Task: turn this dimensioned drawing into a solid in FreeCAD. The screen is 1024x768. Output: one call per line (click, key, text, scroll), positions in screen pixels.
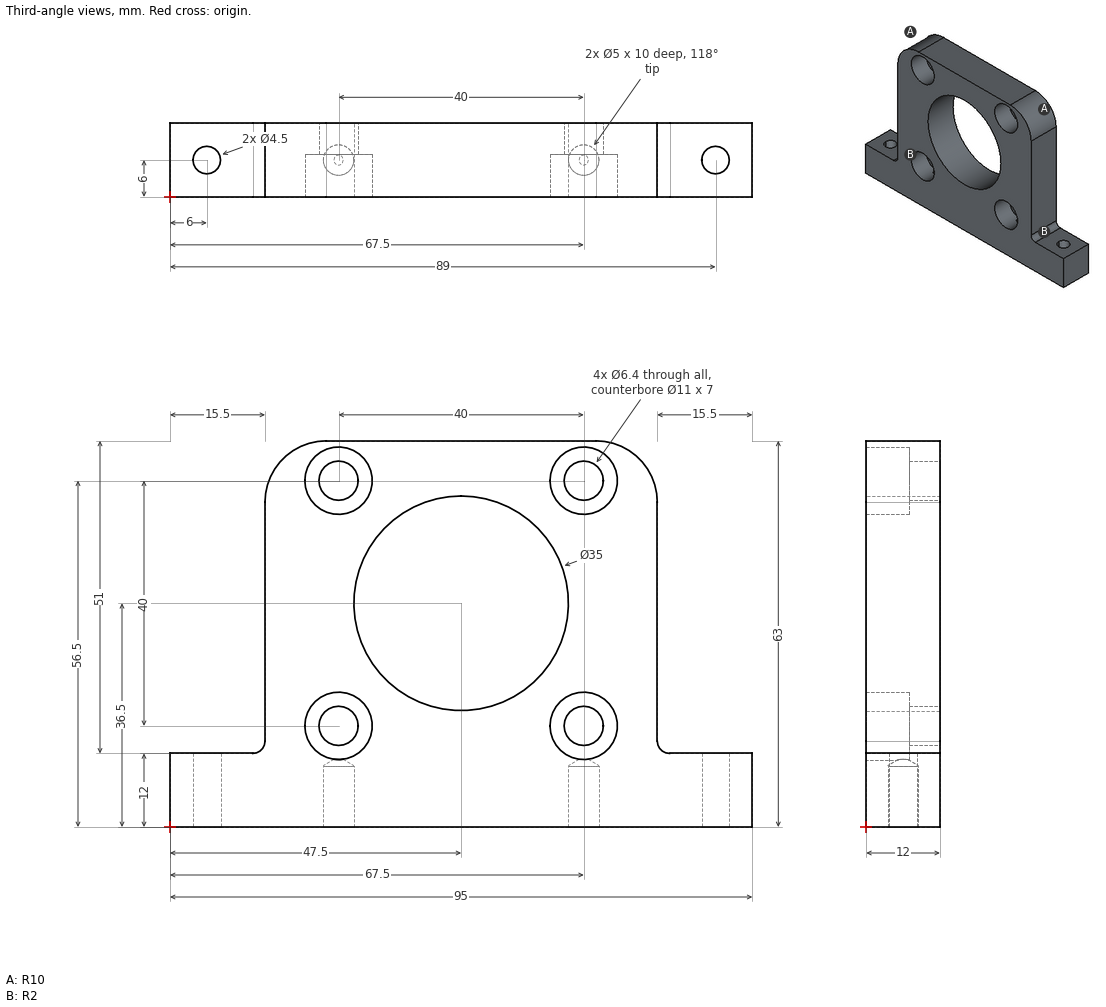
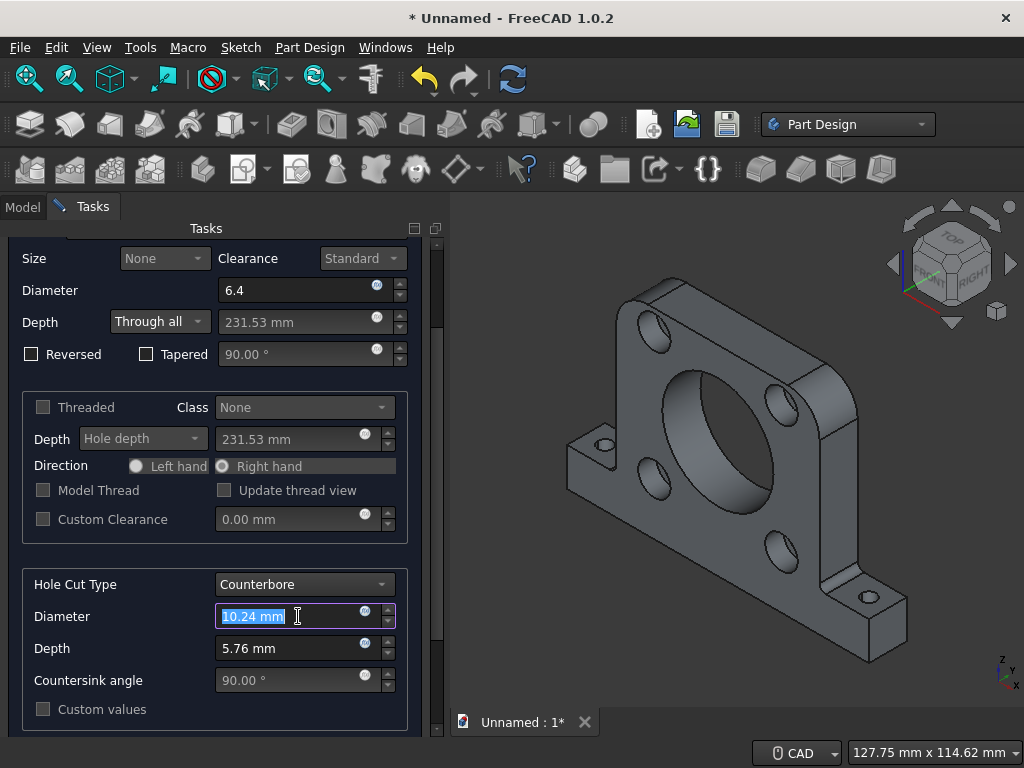
text(11)
key(Tab)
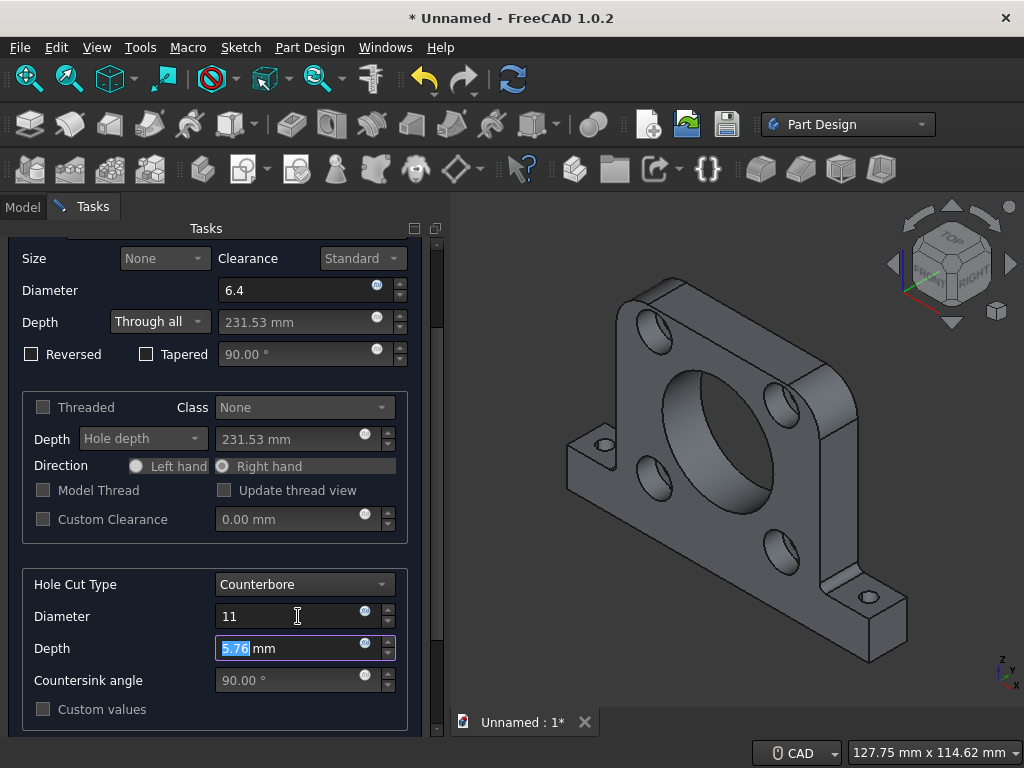
text(7)
key(Tab)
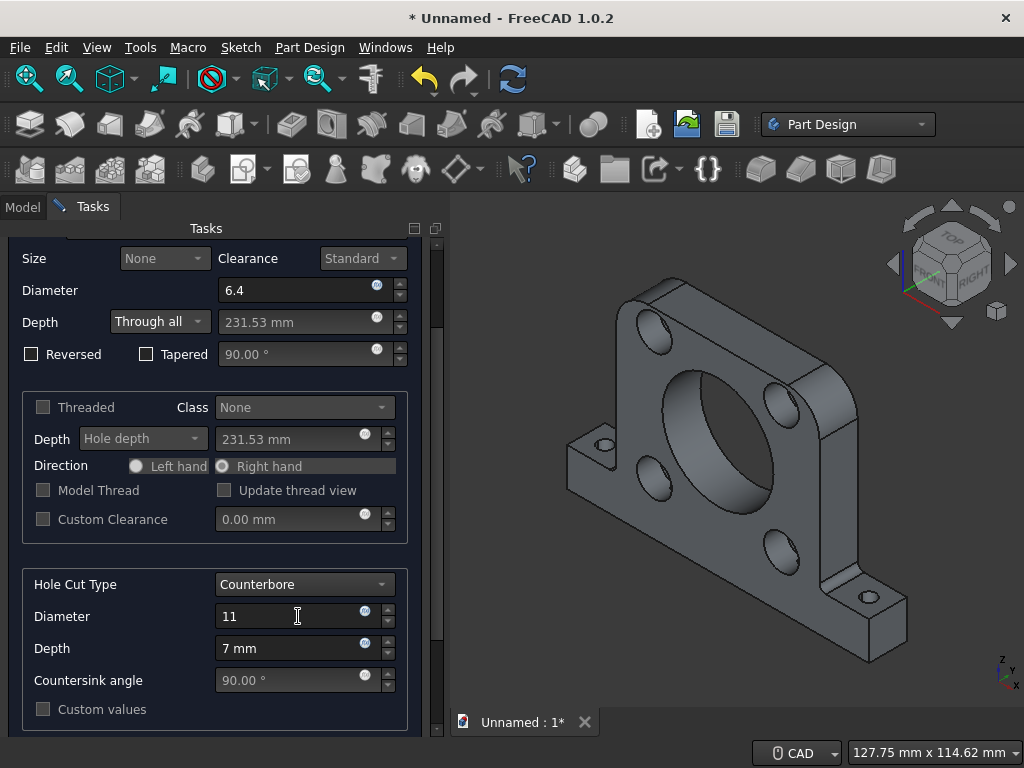
scroll(437, 487, up, 3)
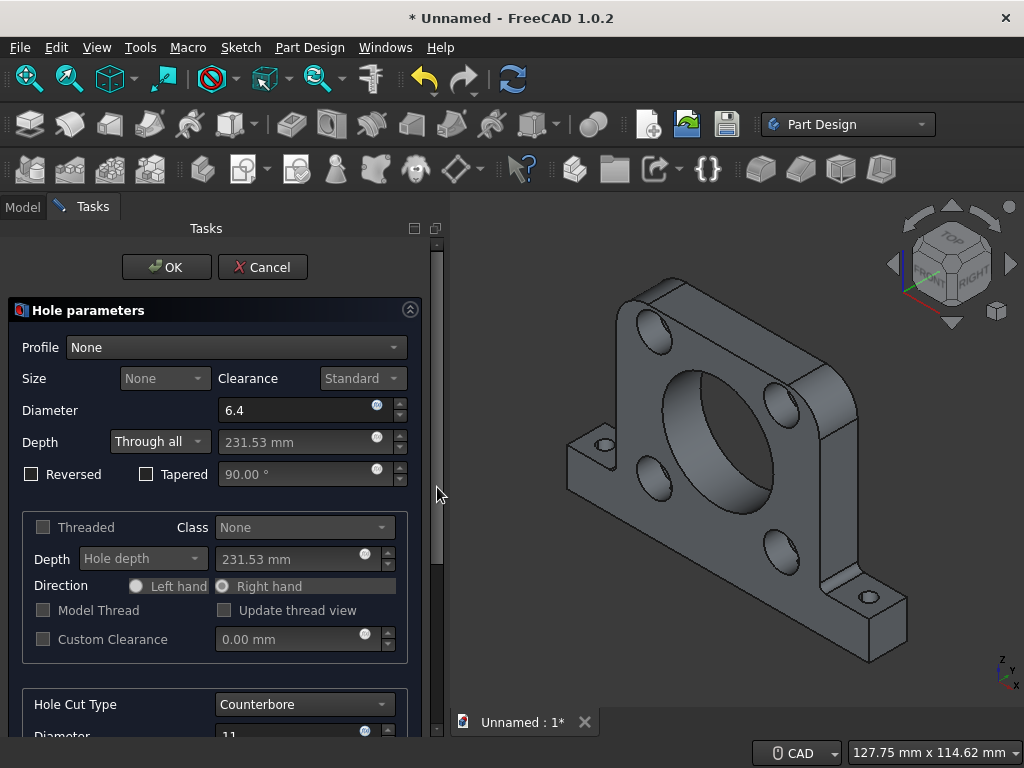
click(167, 267)